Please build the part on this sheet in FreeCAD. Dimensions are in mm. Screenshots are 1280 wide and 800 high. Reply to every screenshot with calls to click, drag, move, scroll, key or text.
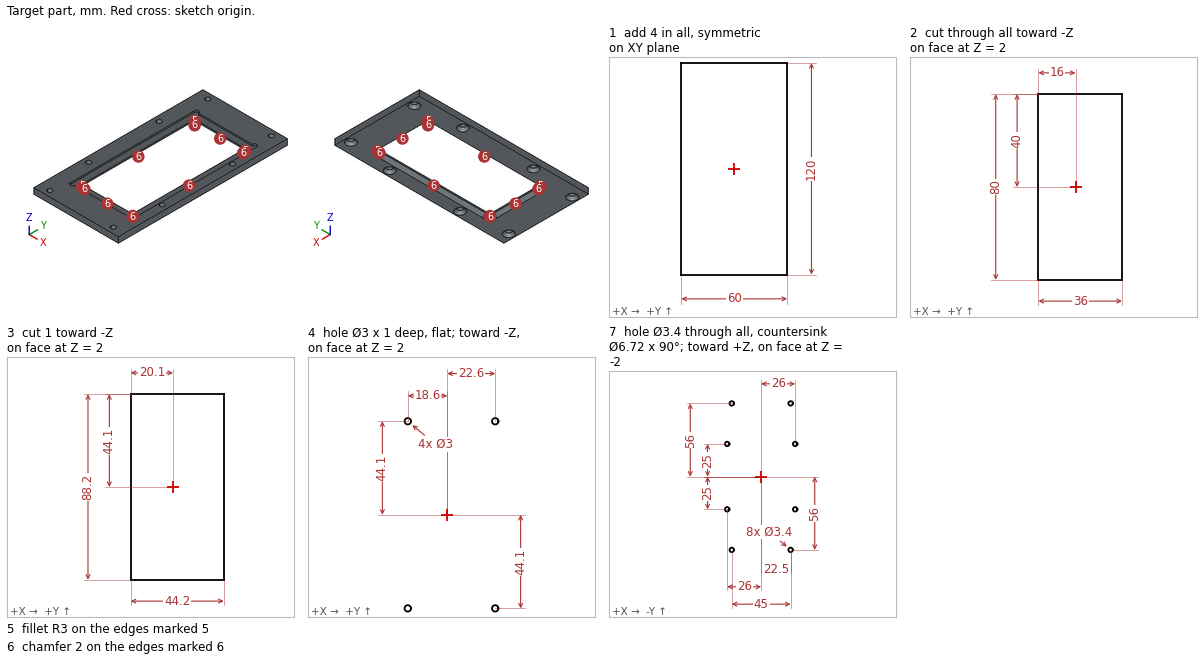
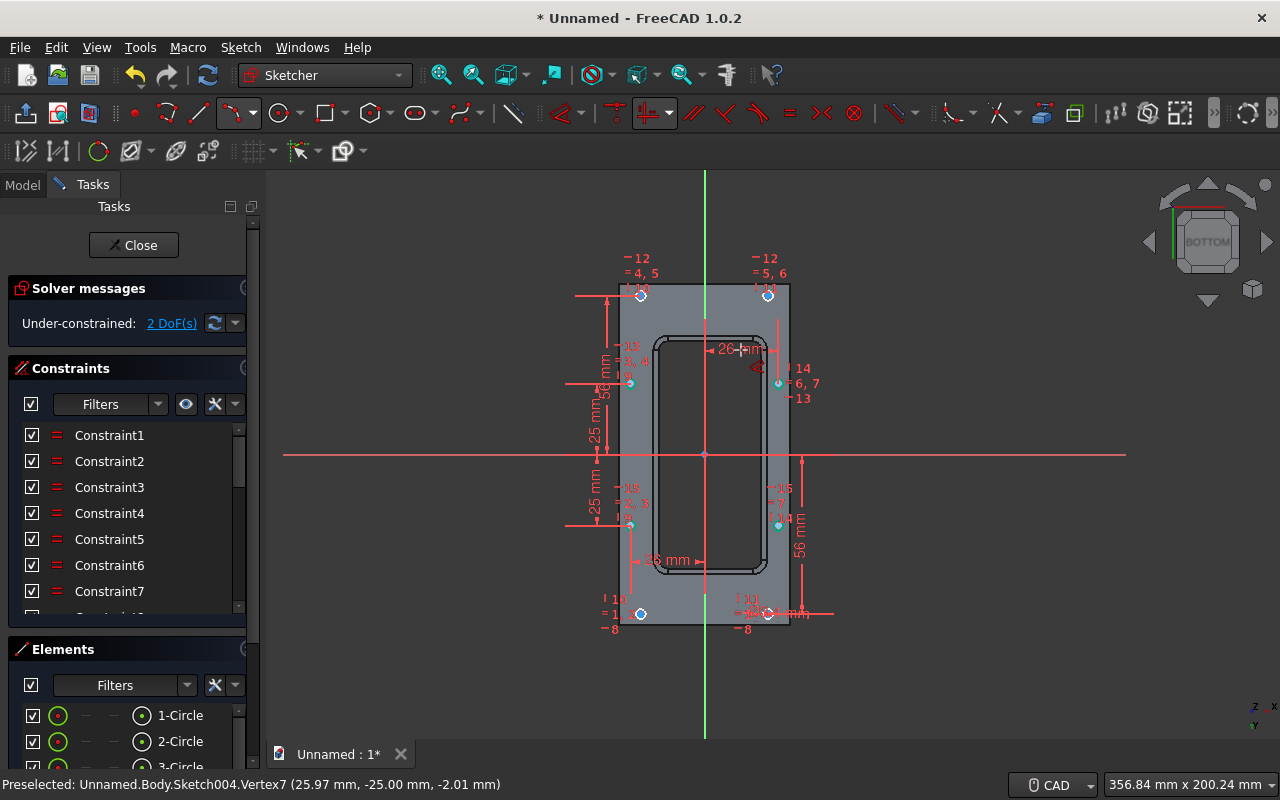
click(768, 614)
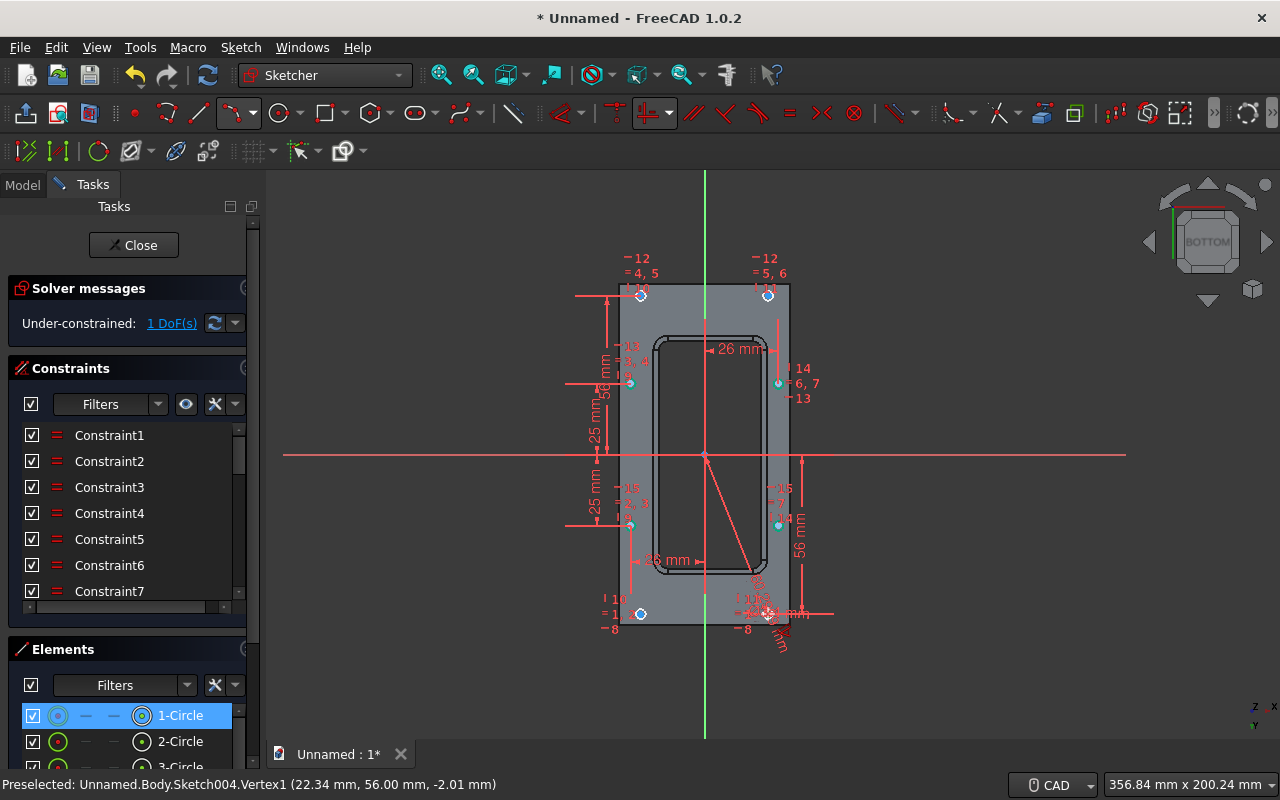
click(641, 614)
click(675, 648)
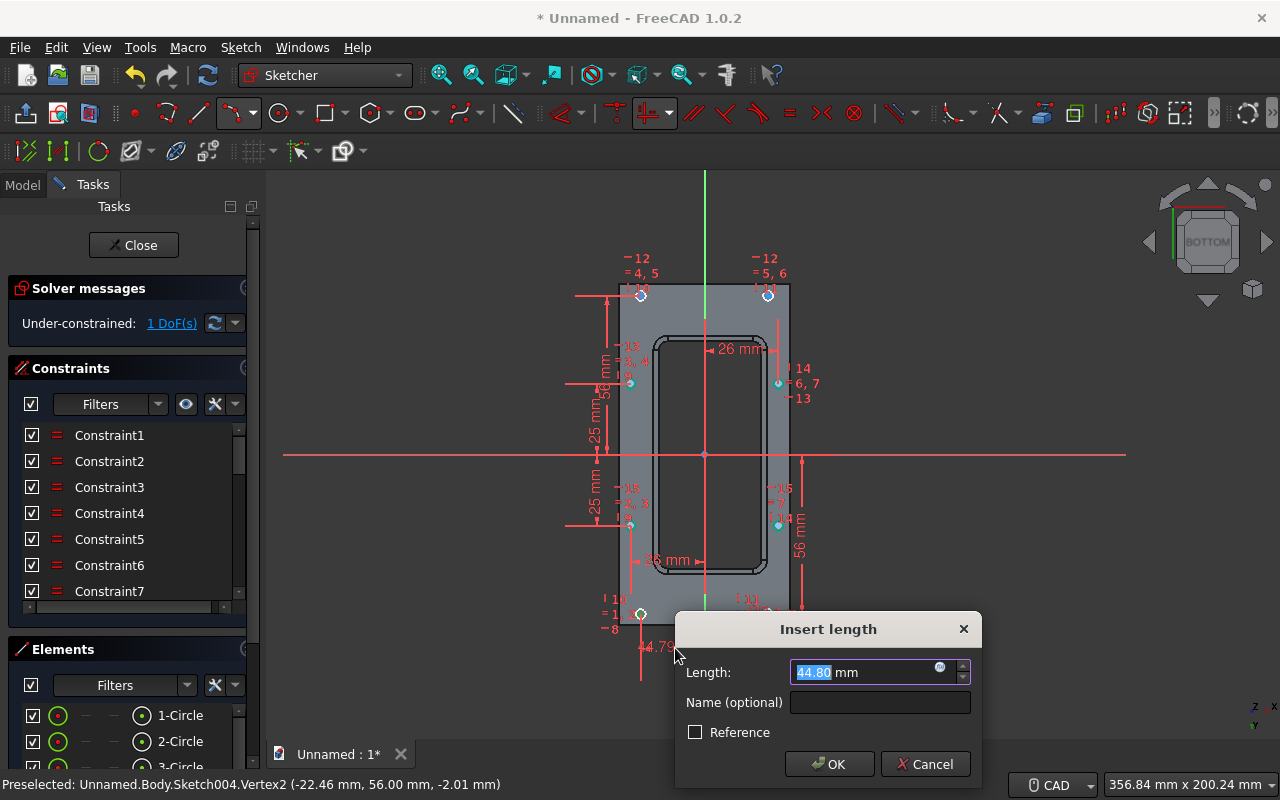
text(45)
key(Return)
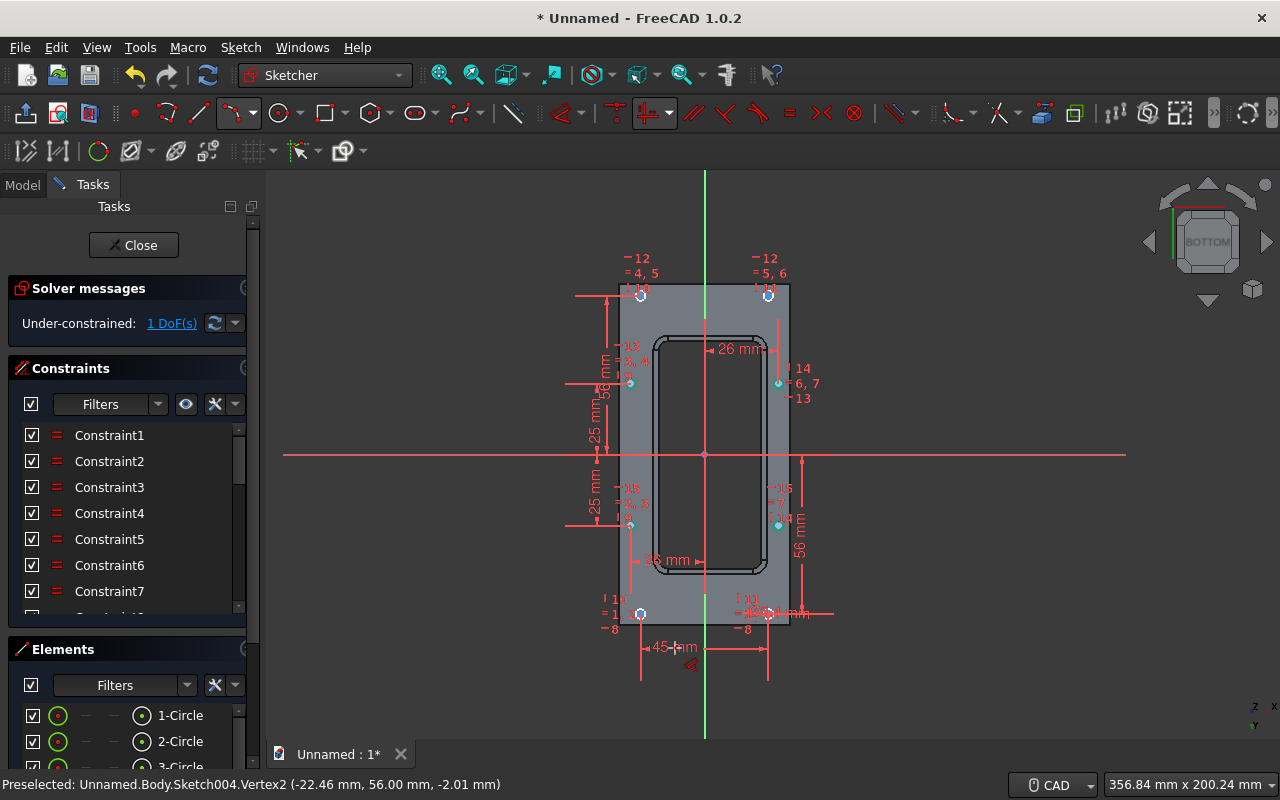
click(768, 614)
click(751, 648)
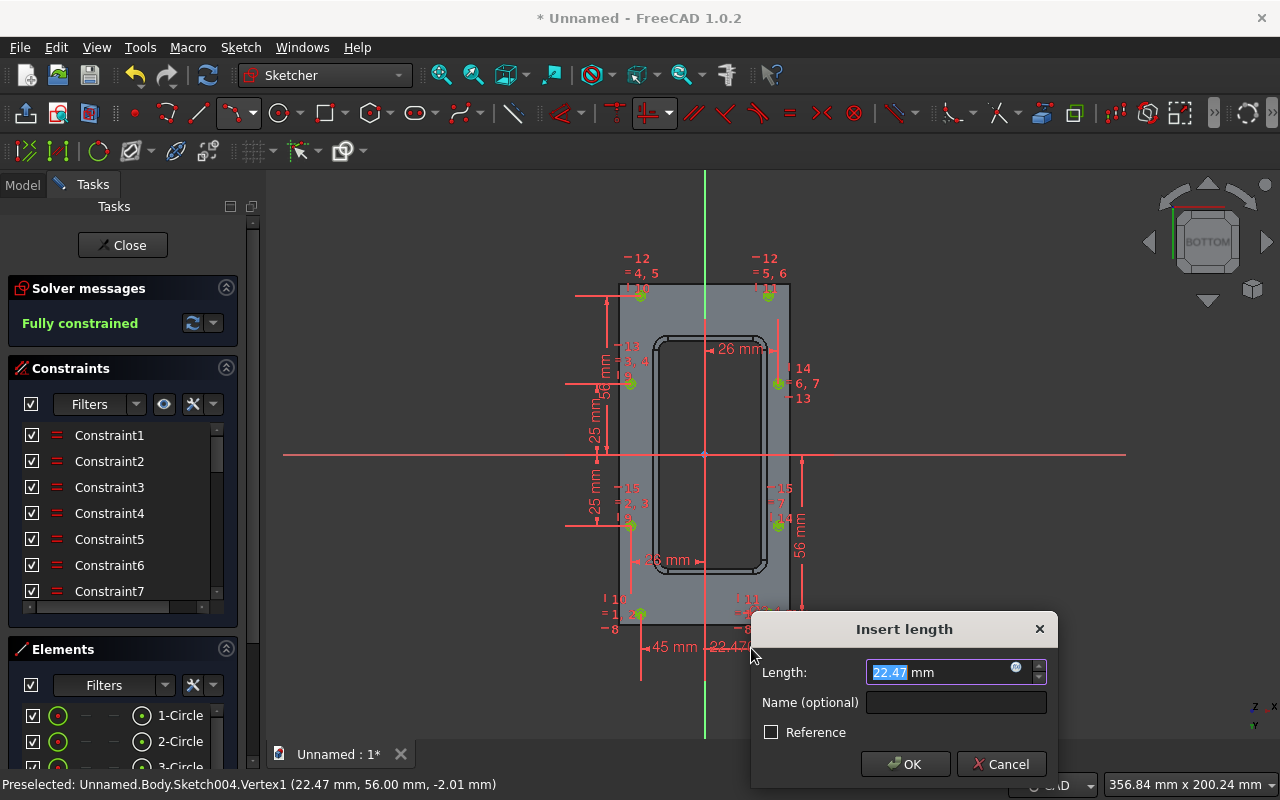
text(22.5)
key(Return)
key(Escape)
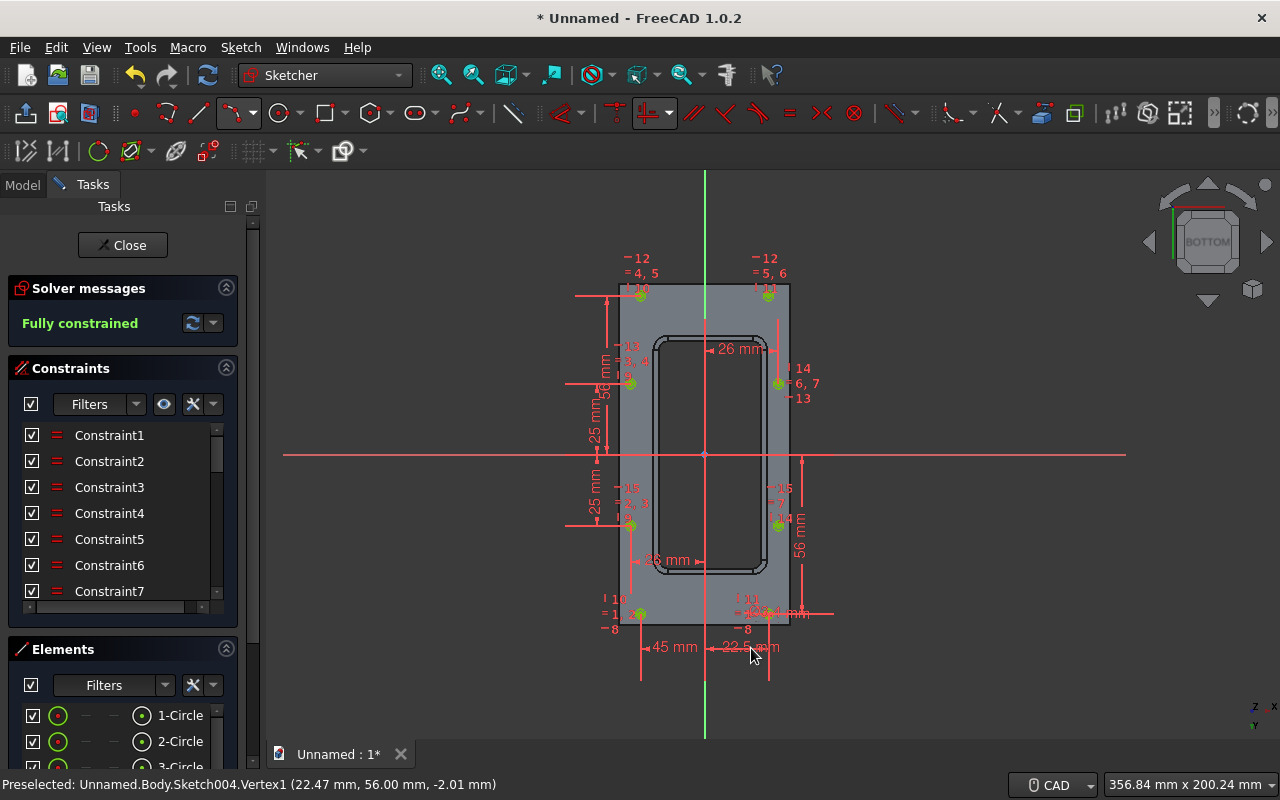
click(123, 245)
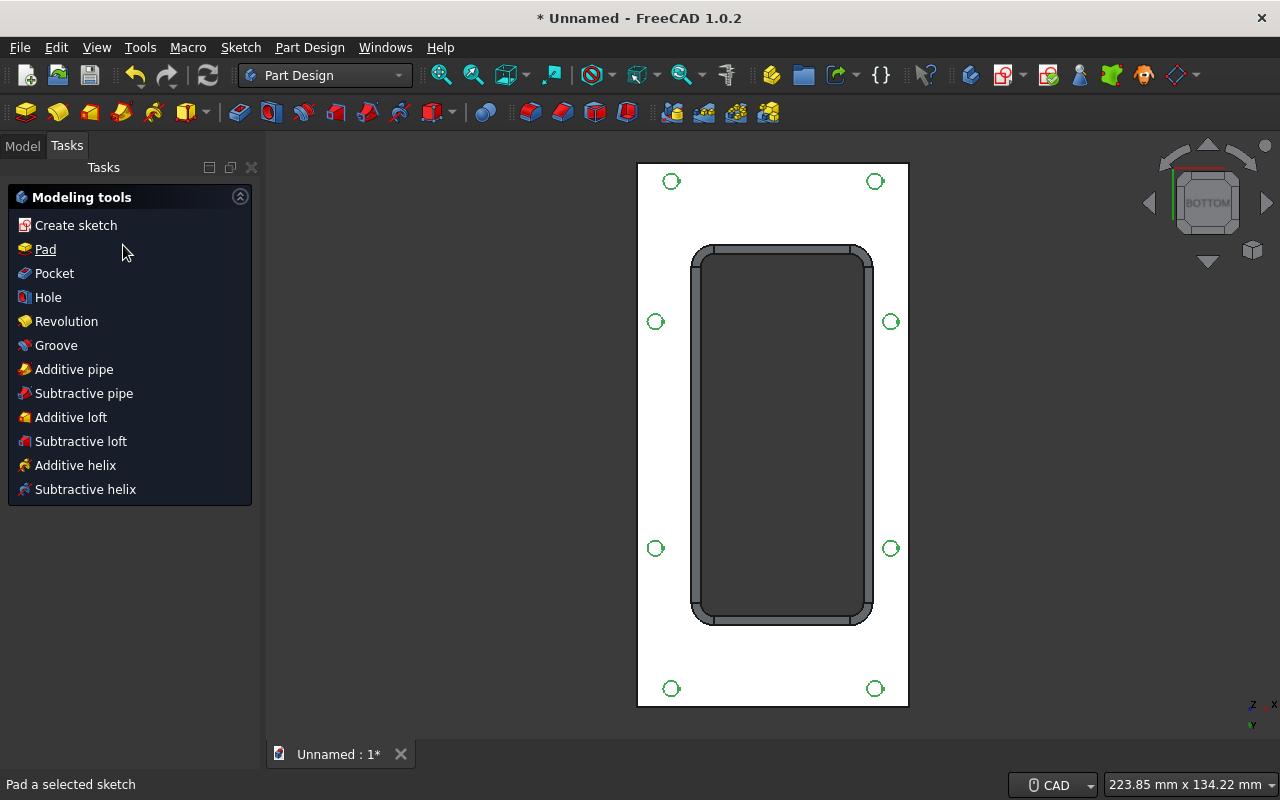
click(272, 112)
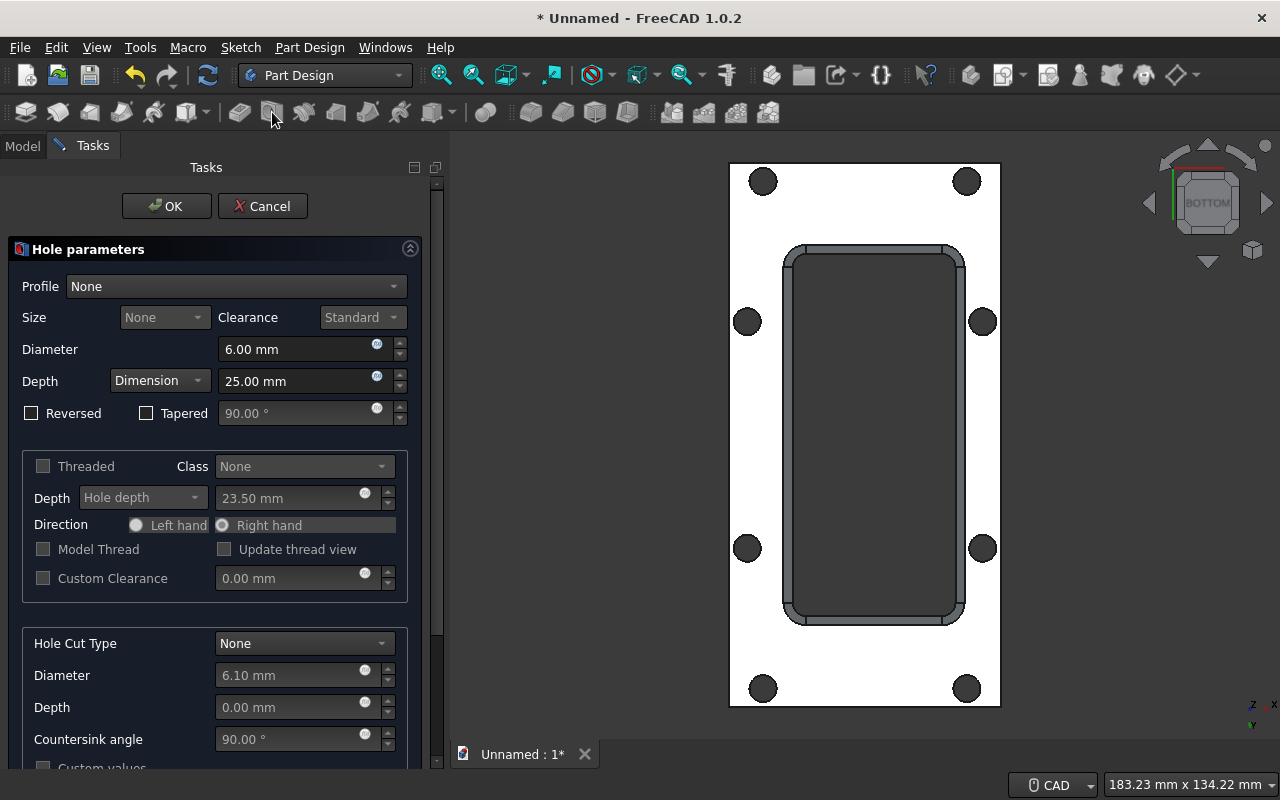
triple_click(305, 349)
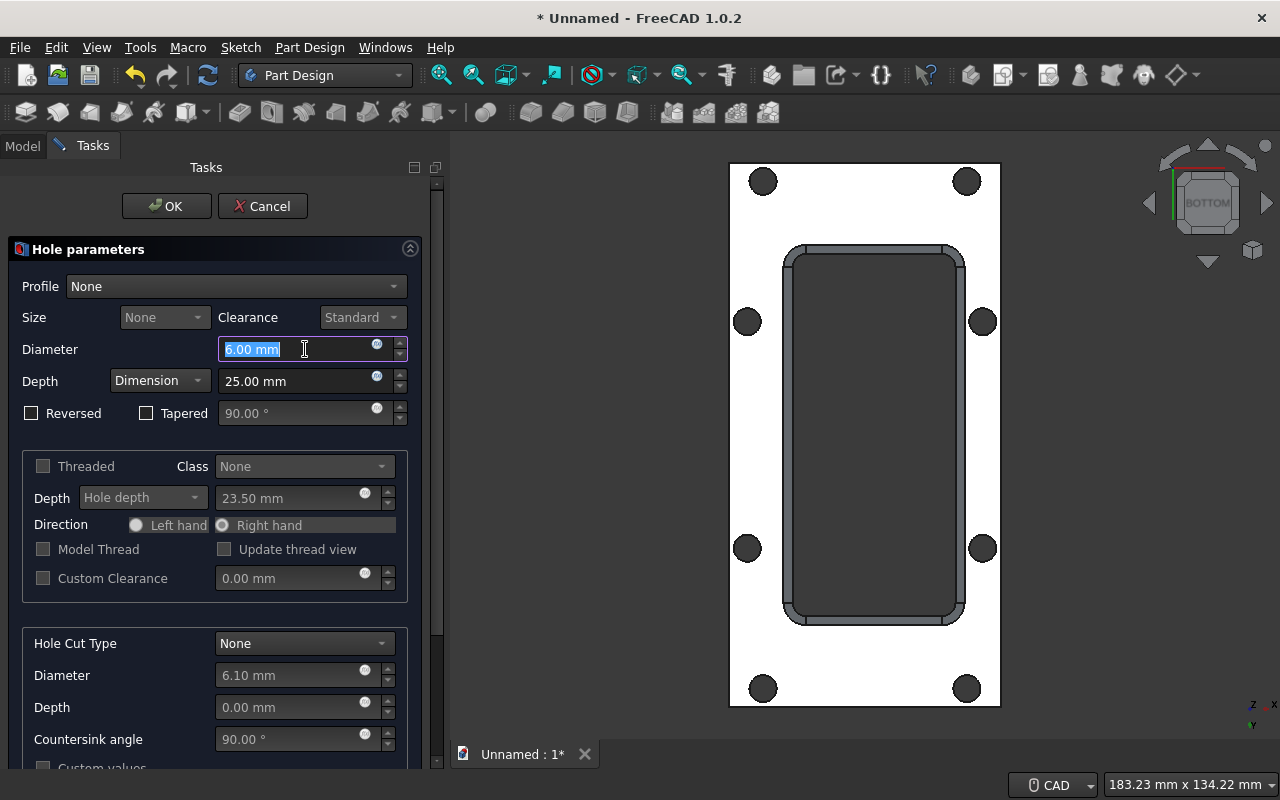
text(3.4)
key(Tab)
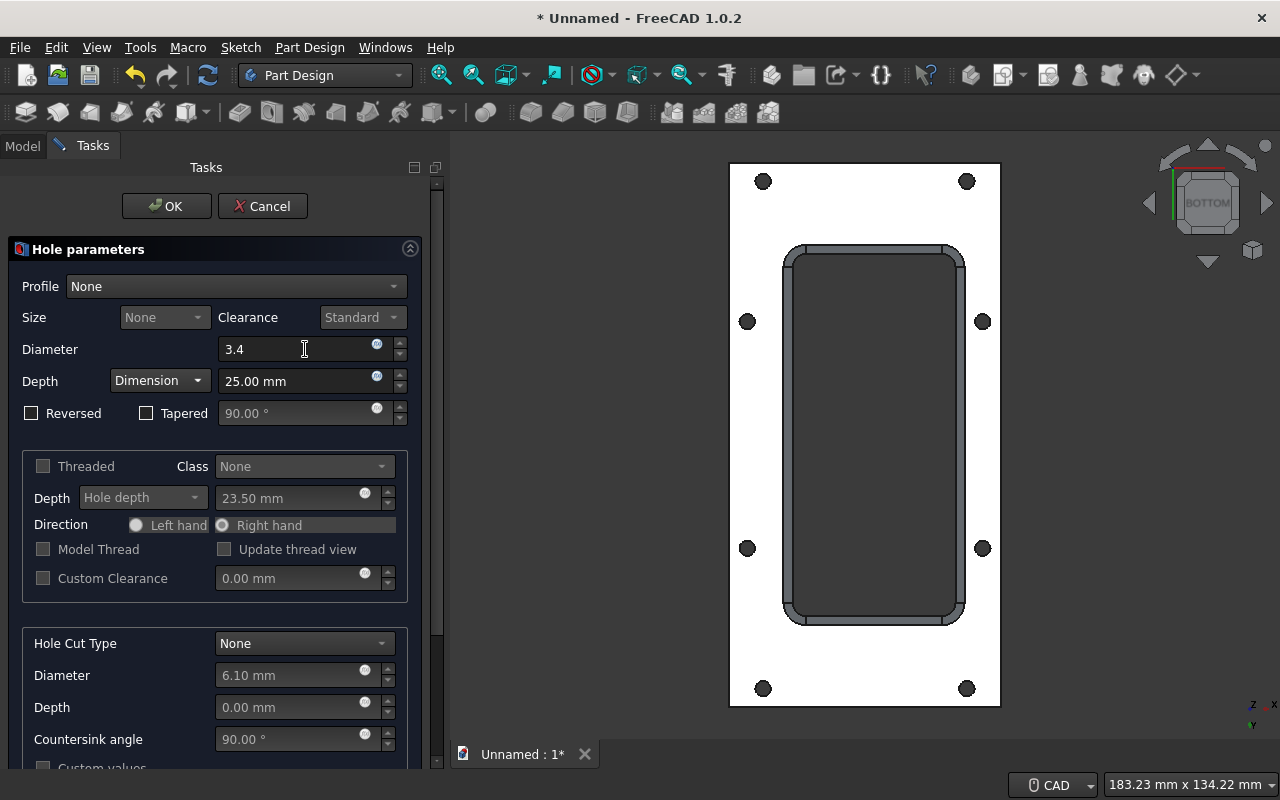
click(161, 380)